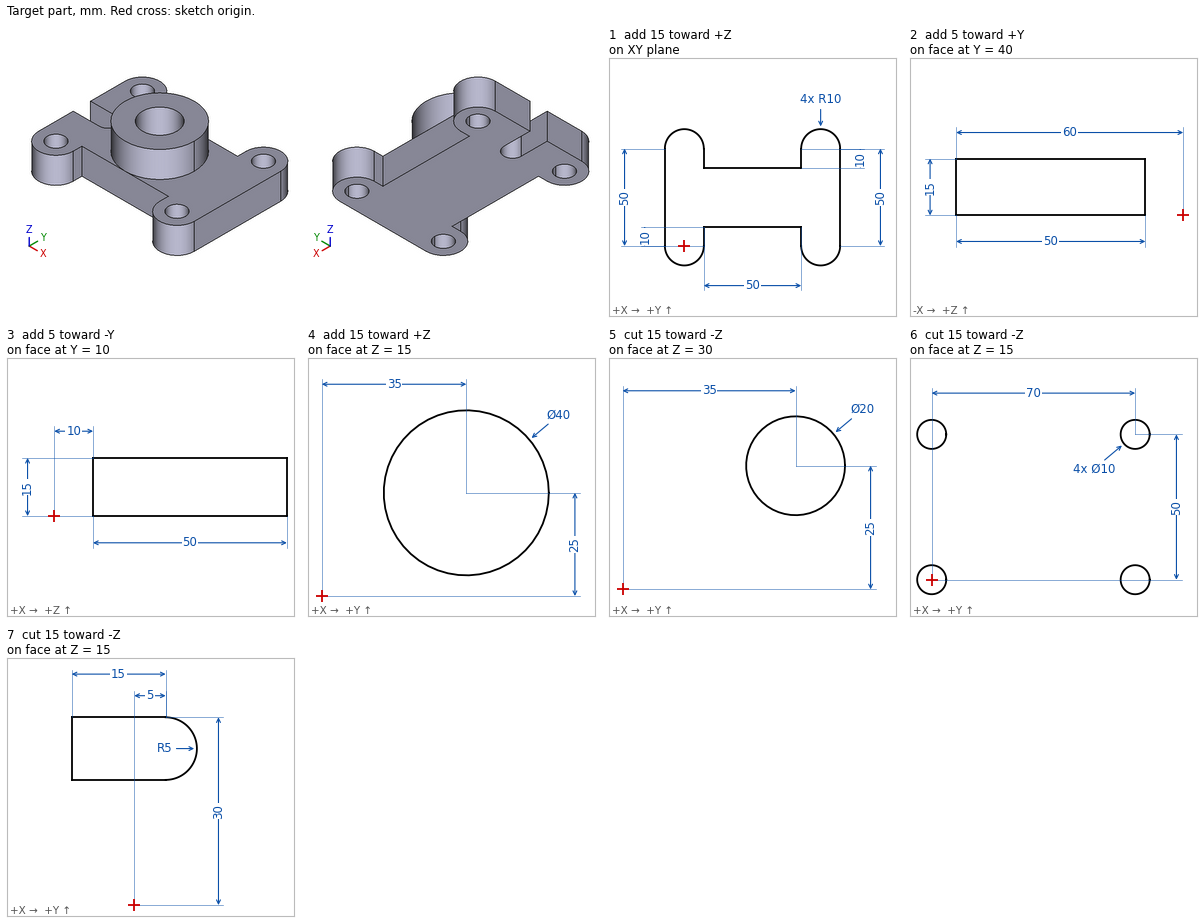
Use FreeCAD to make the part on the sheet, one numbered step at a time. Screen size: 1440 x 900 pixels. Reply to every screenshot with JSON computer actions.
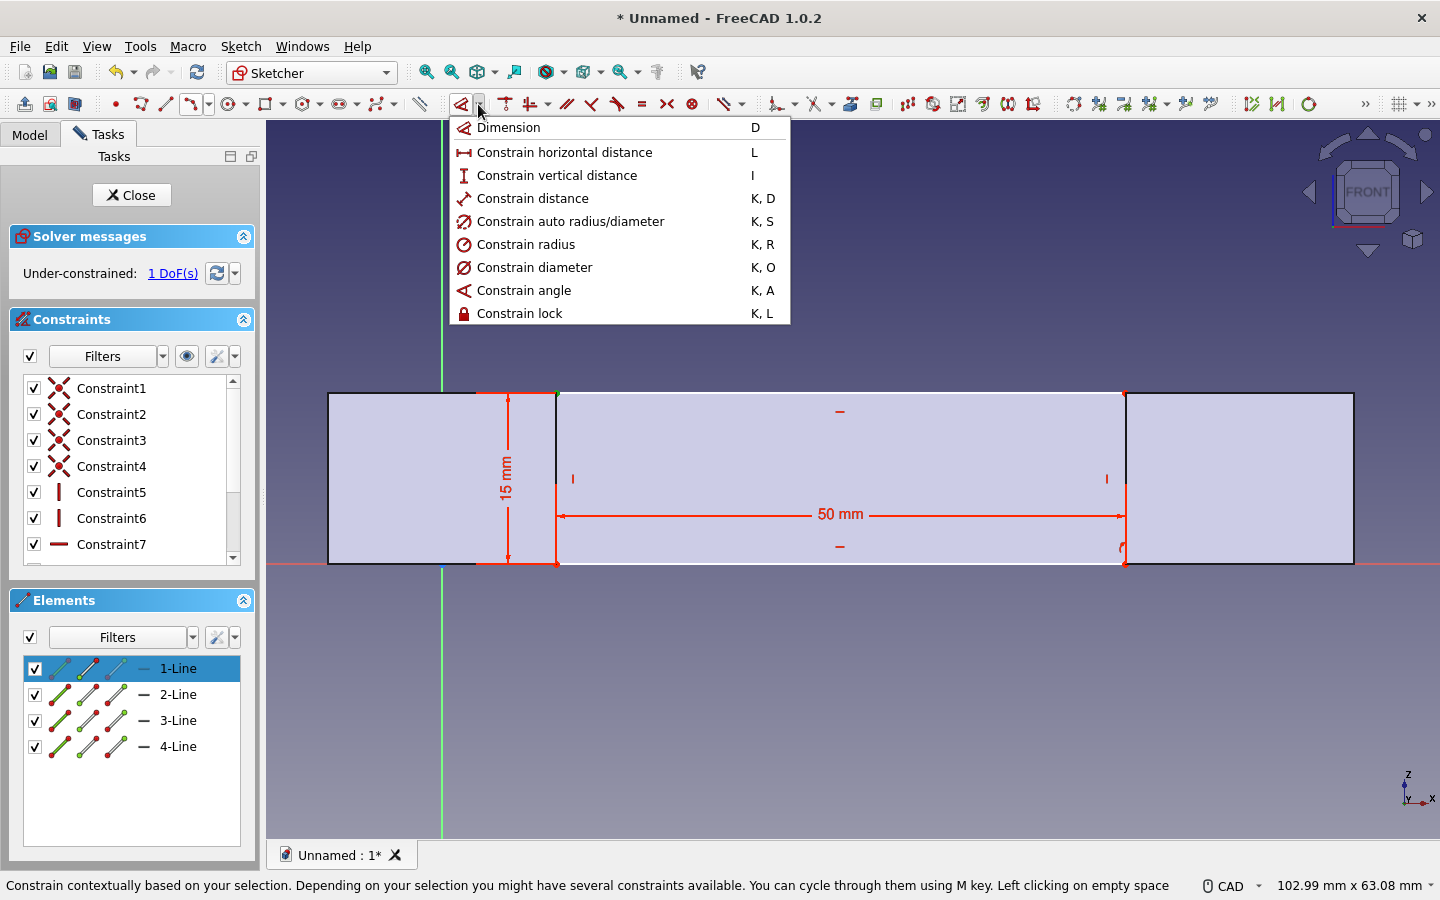
{"action": "left_click", "coordinate": [620, 152]}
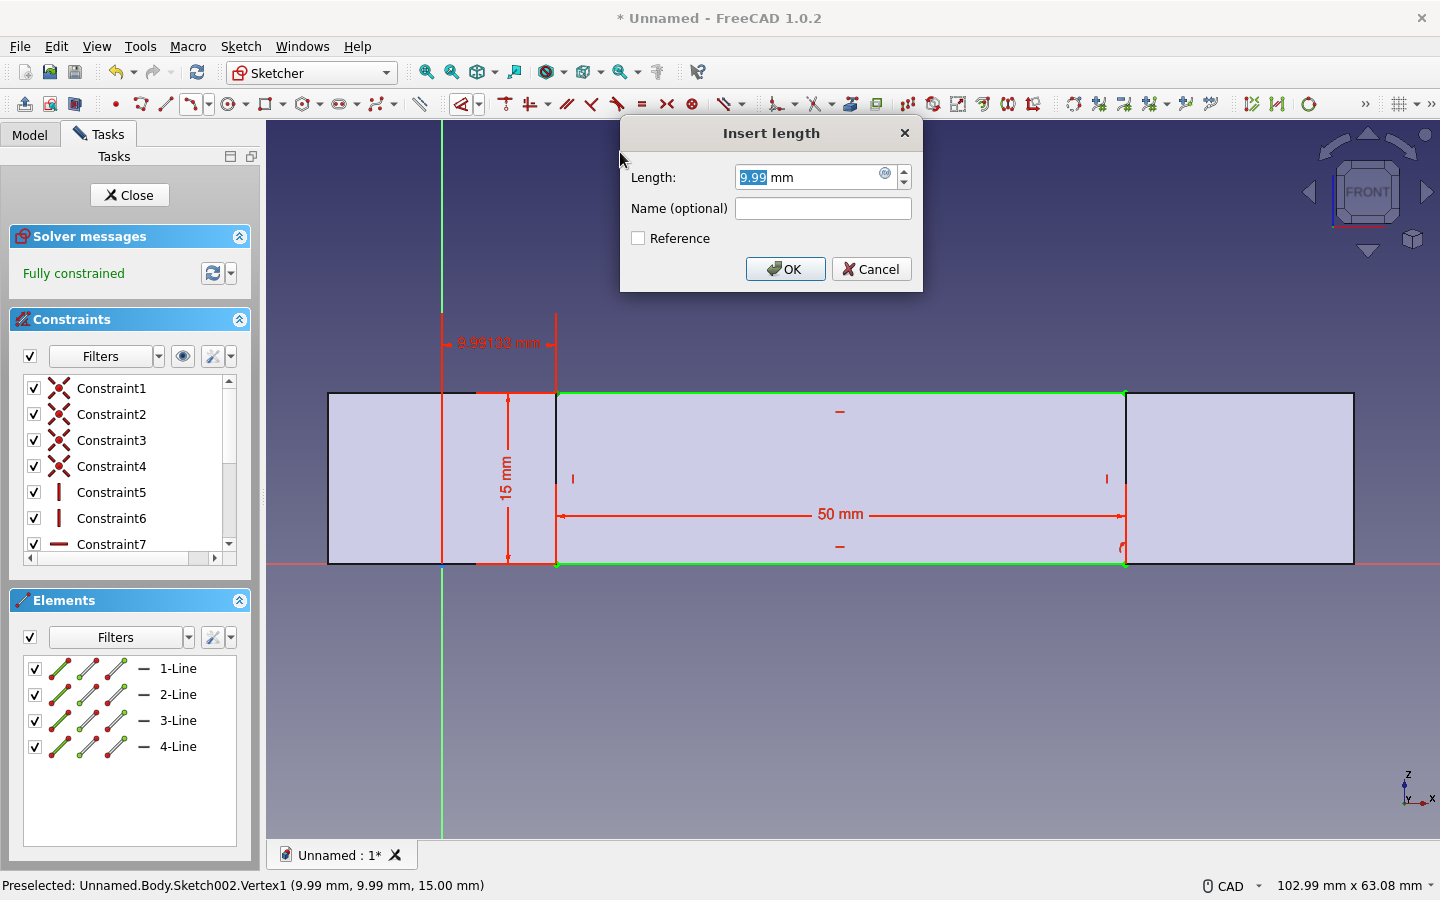
{"action": "type", "text": "10"}
{"action": "key", "text": "Return"}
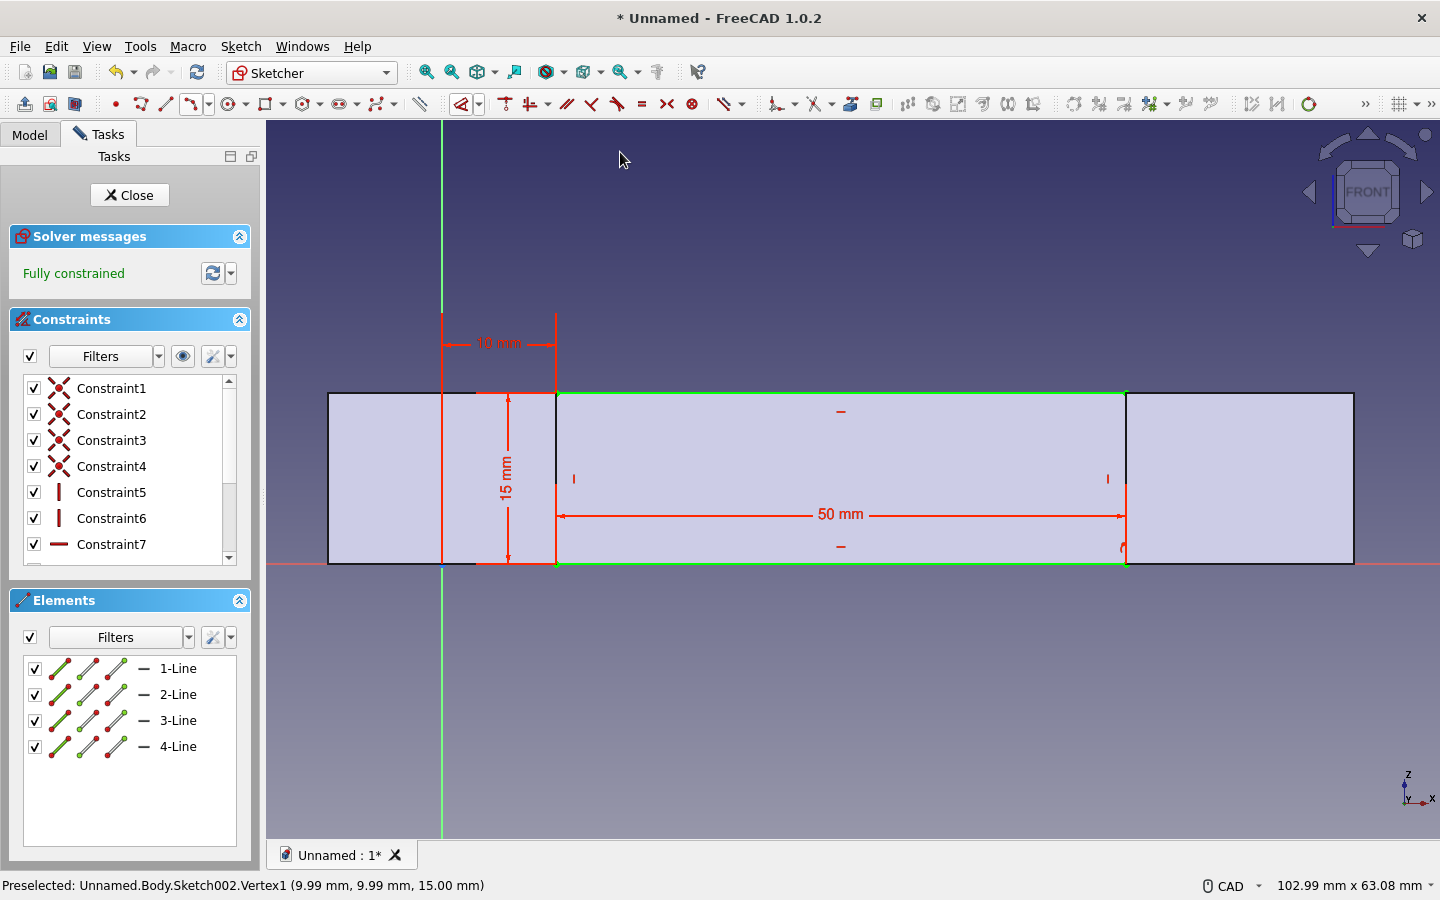
{"action": "left_click", "coordinate": [130, 195]}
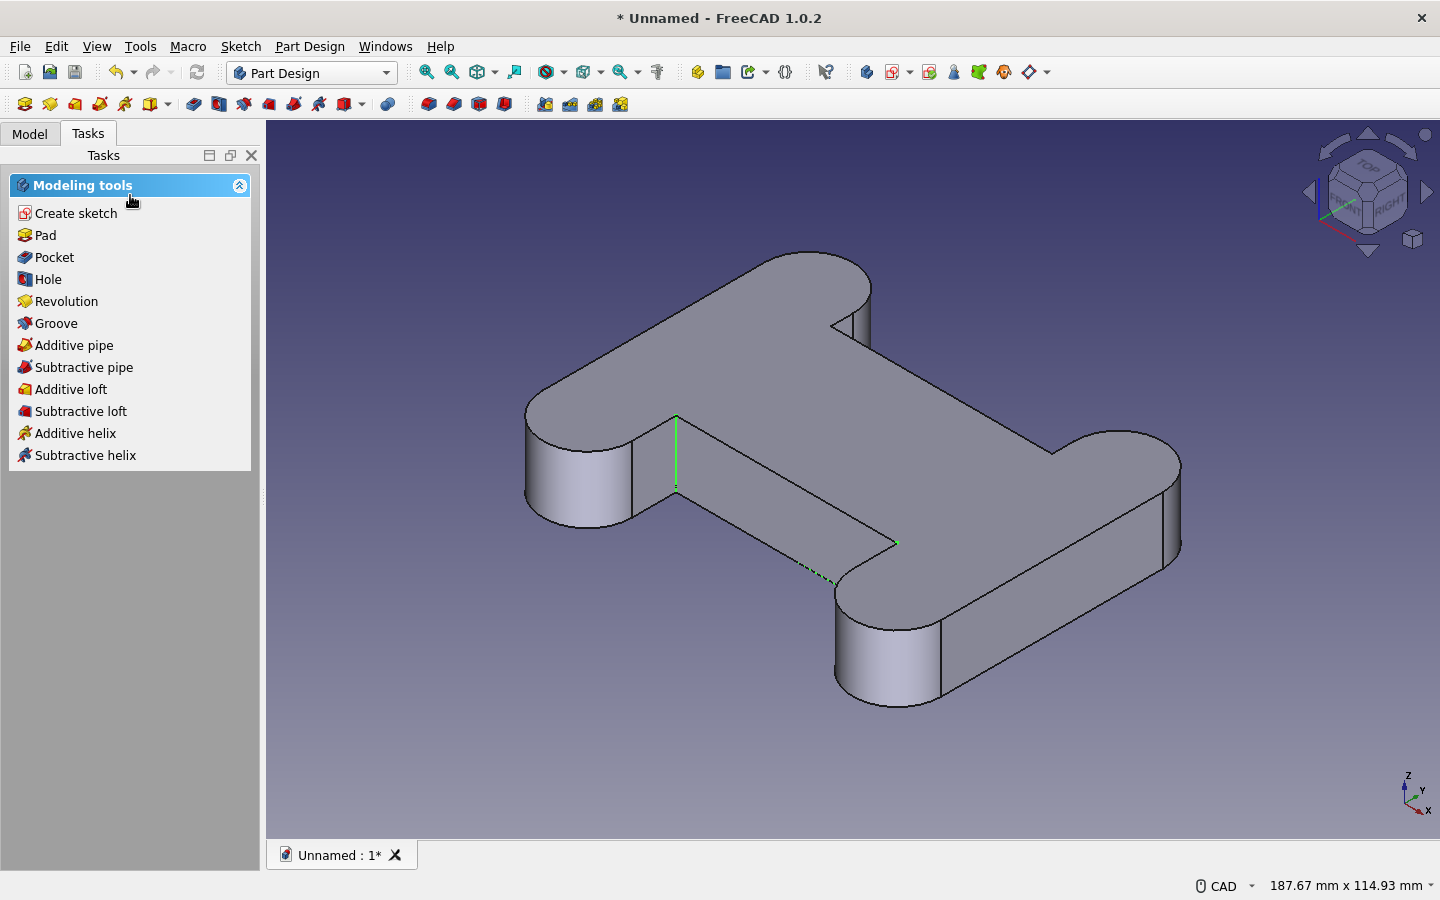
{"action": "left_click", "coordinate": [25, 104]}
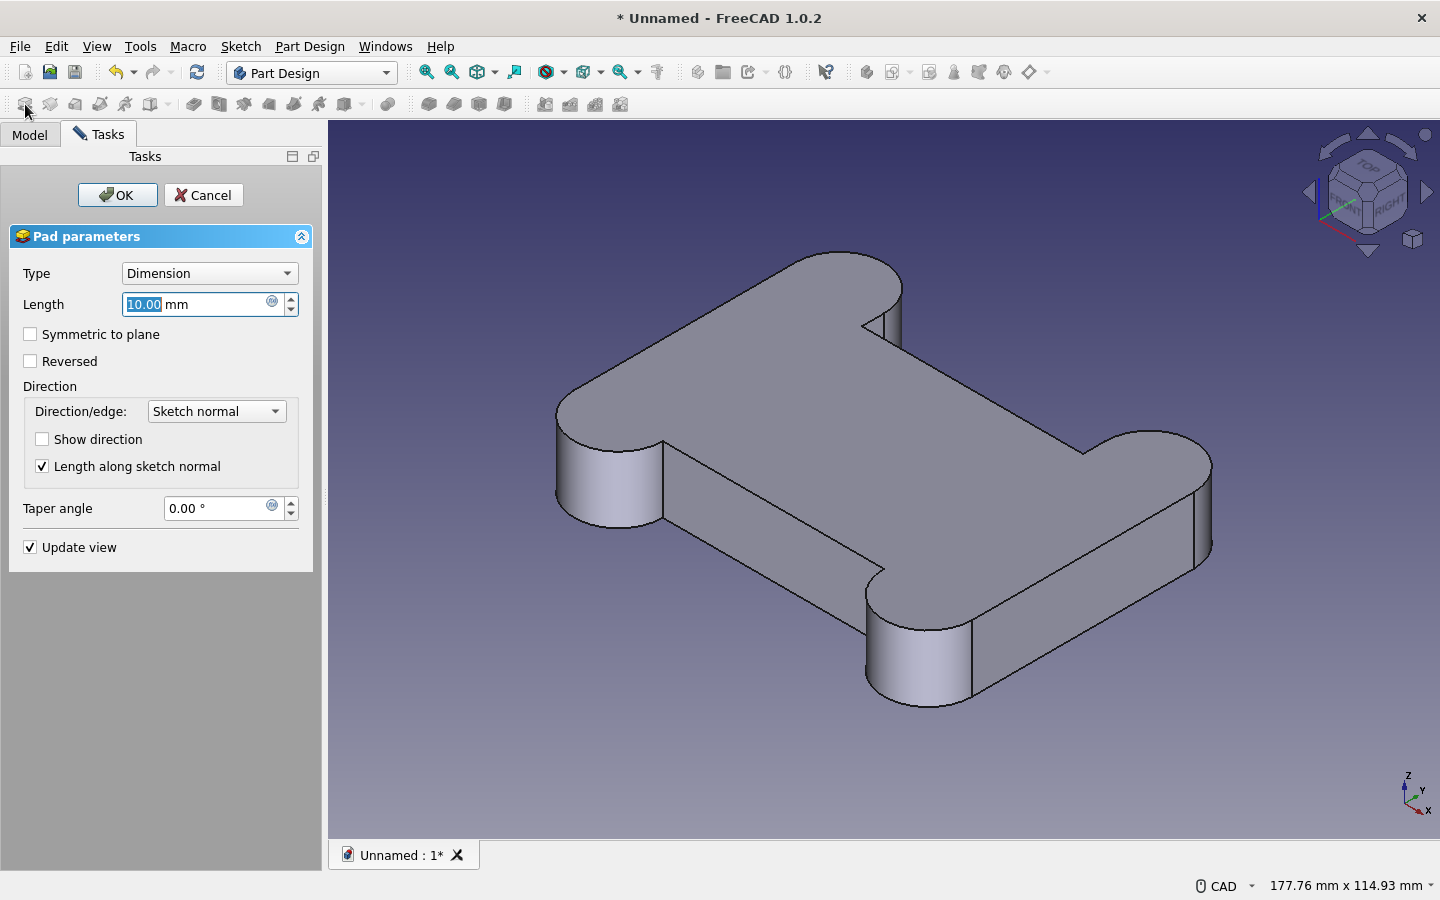
{"action": "type", "text": "5"}
{"action": "key", "text": "Tab"}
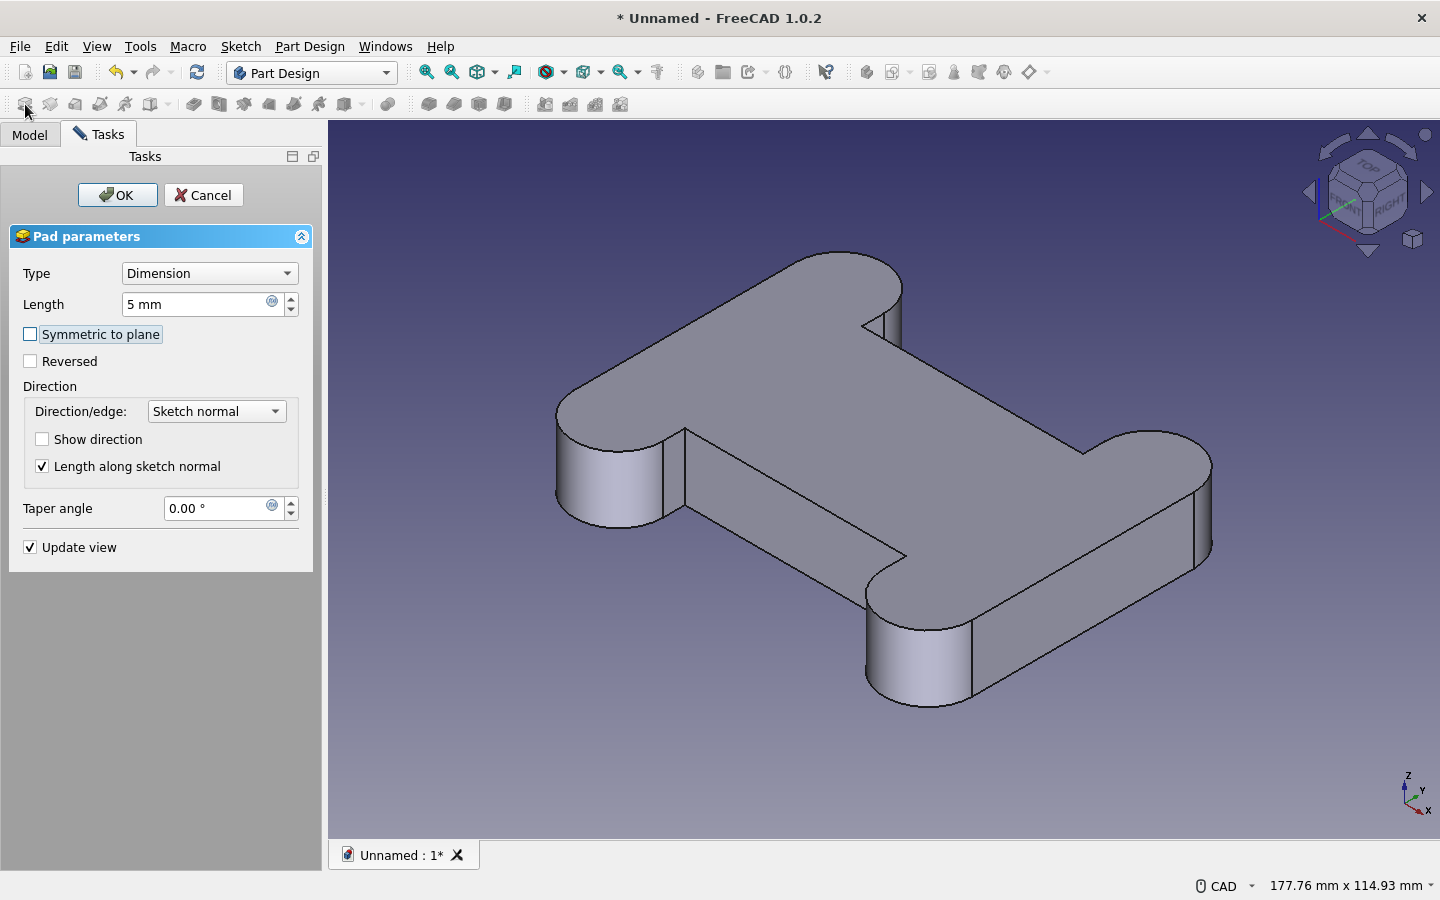
{"action": "left_click", "coordinate": [118, 195]}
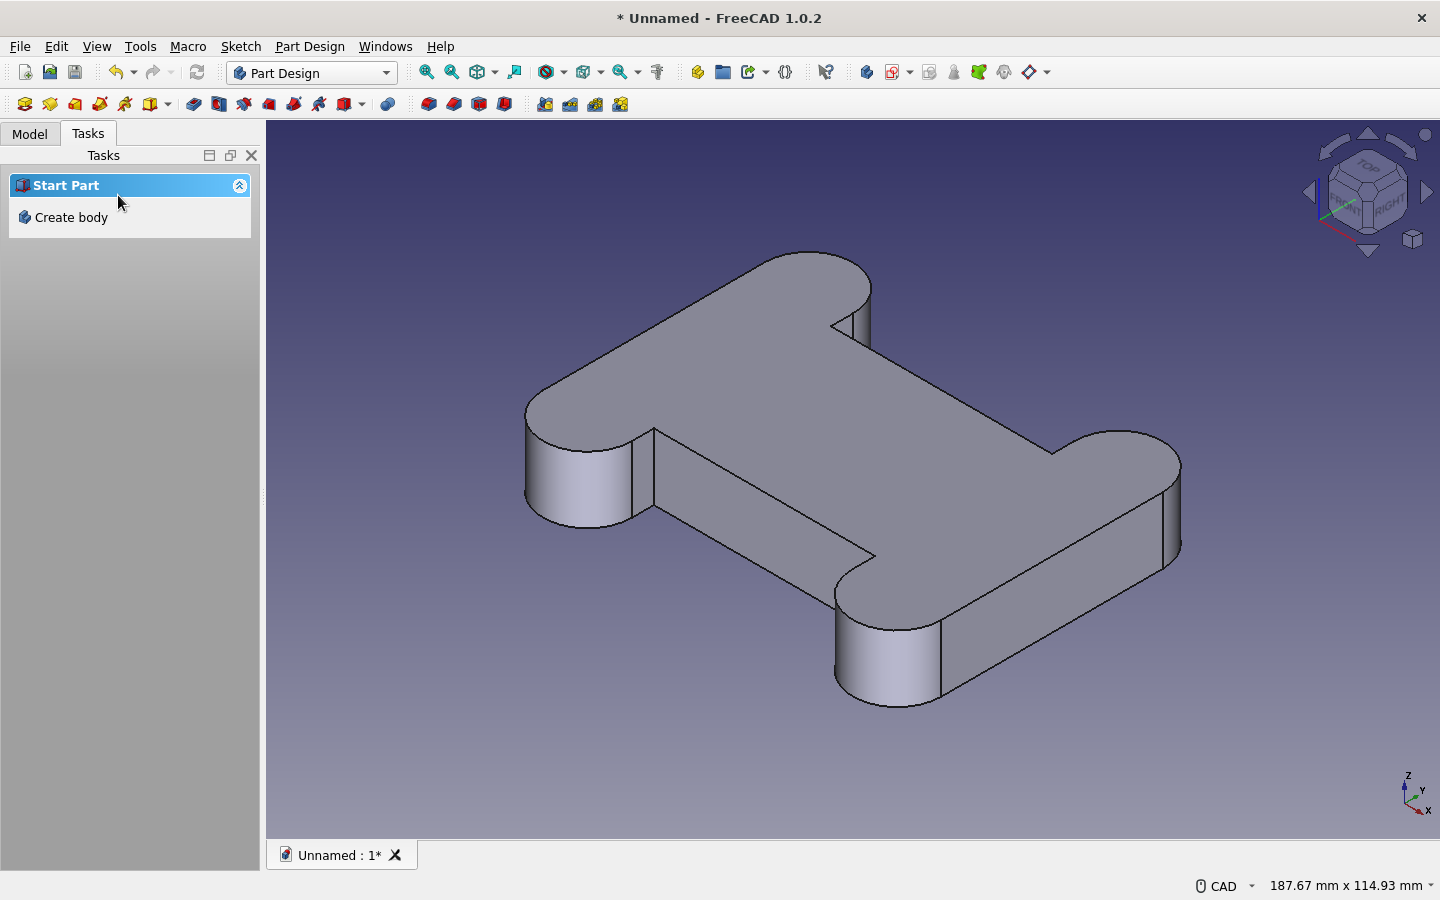
{"action": "left_click", "coordinate": [910, 473]}